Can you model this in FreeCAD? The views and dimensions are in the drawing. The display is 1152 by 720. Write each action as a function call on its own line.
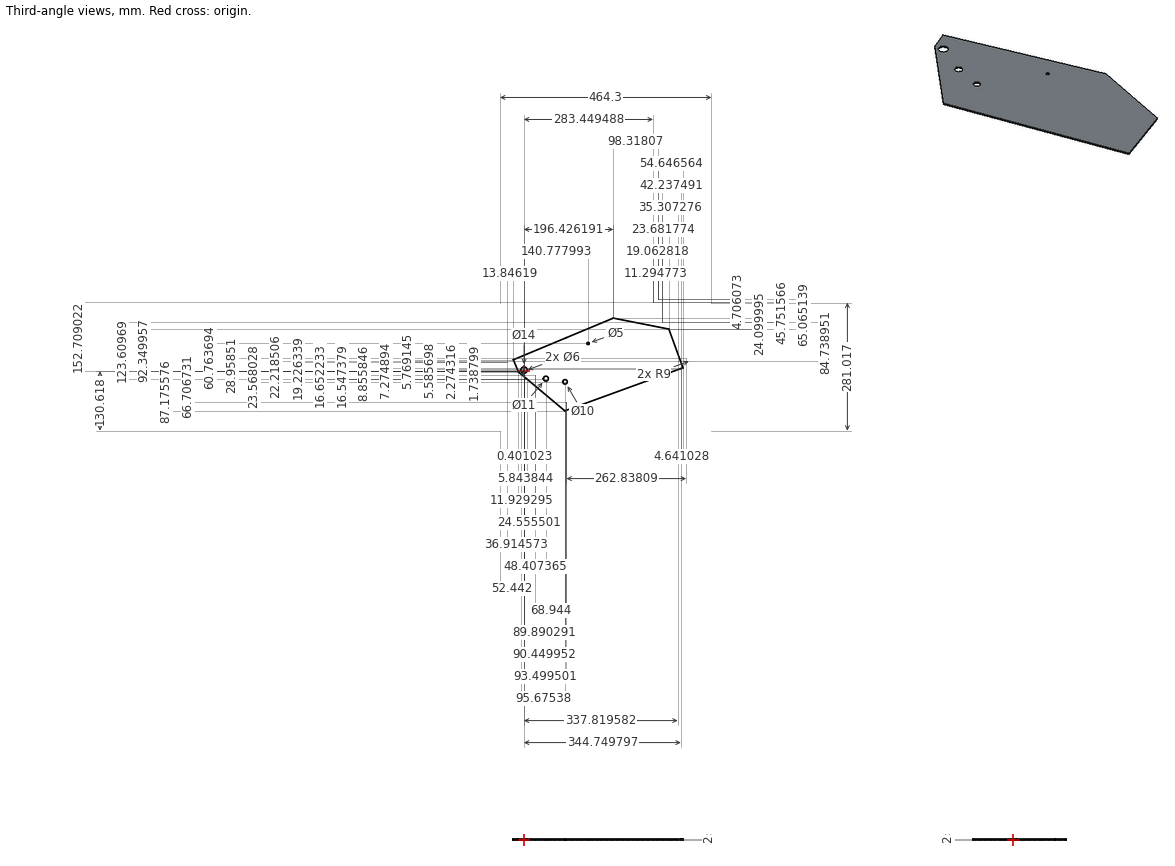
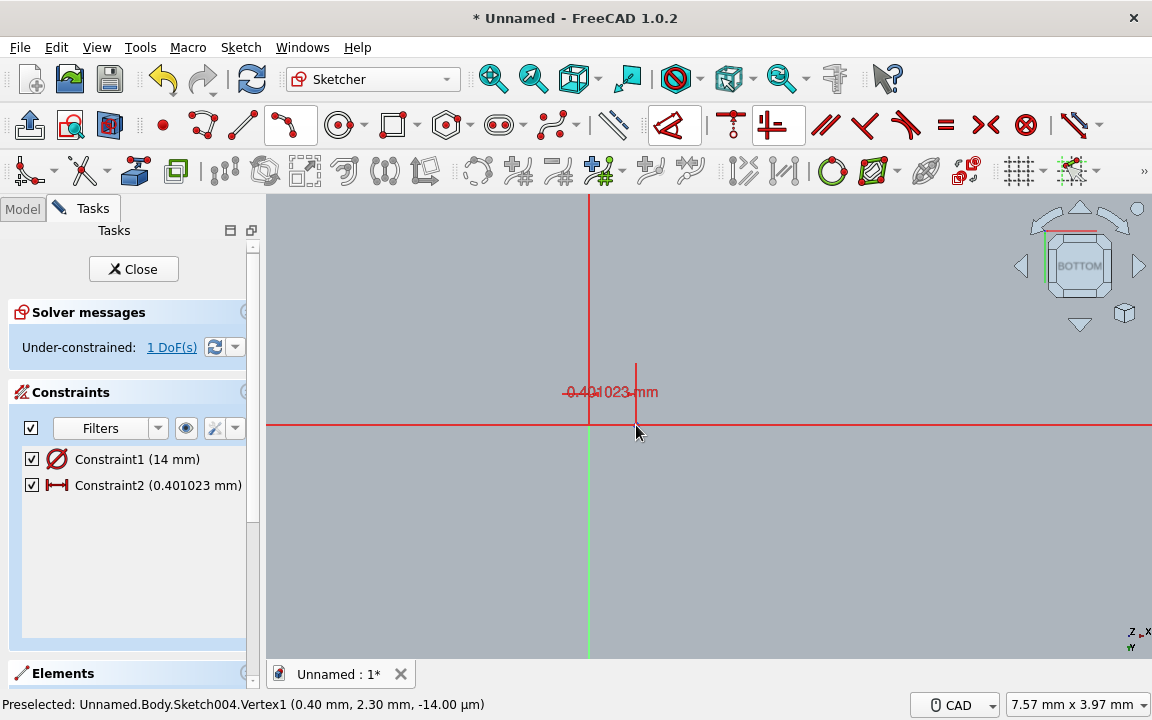
scroll(641, 427, down, 9)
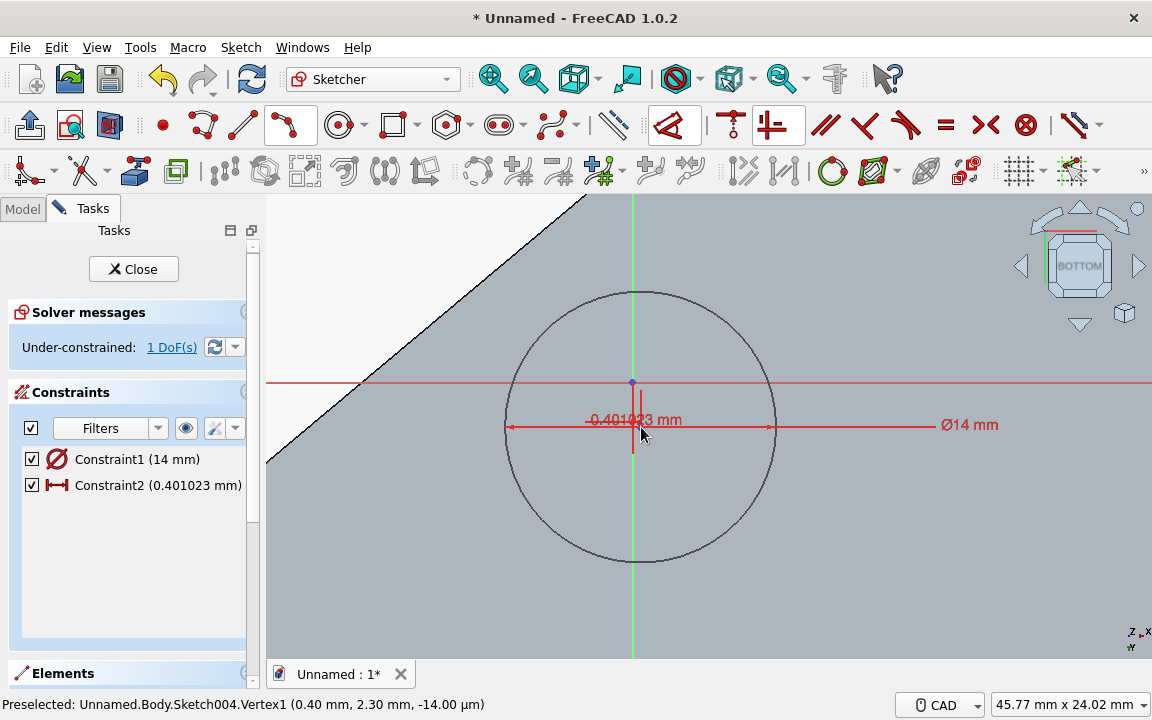
click(641, 427)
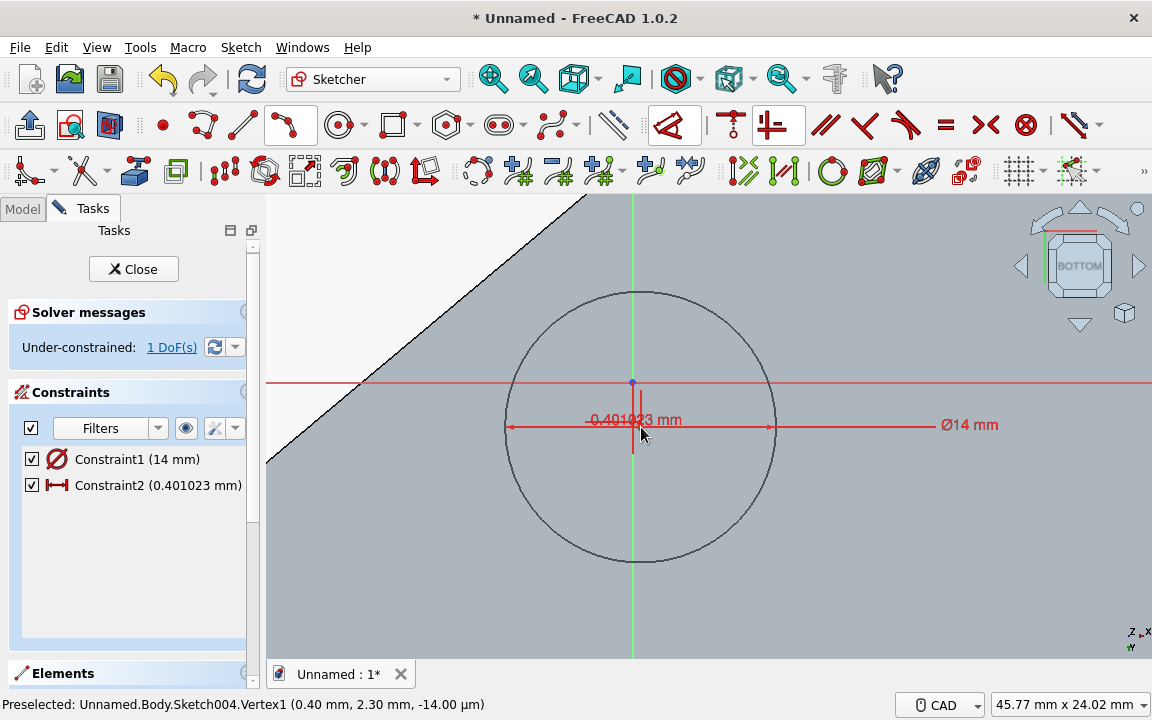
key(i)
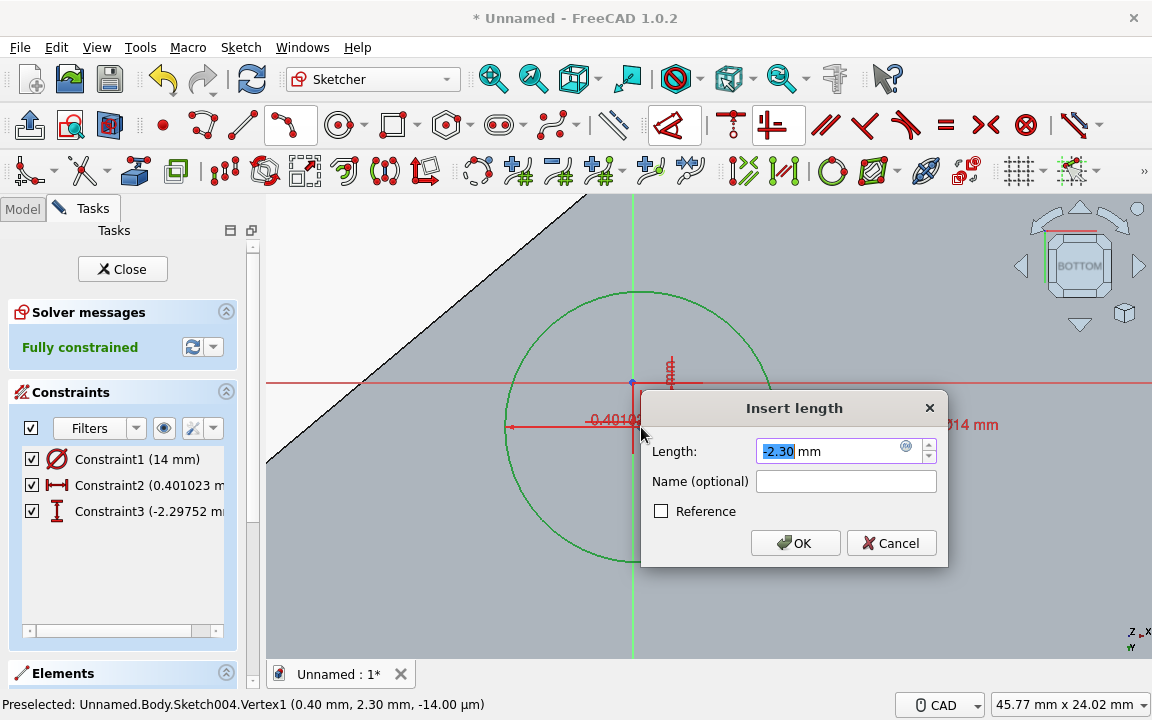
text(-2.274316)
key(Return)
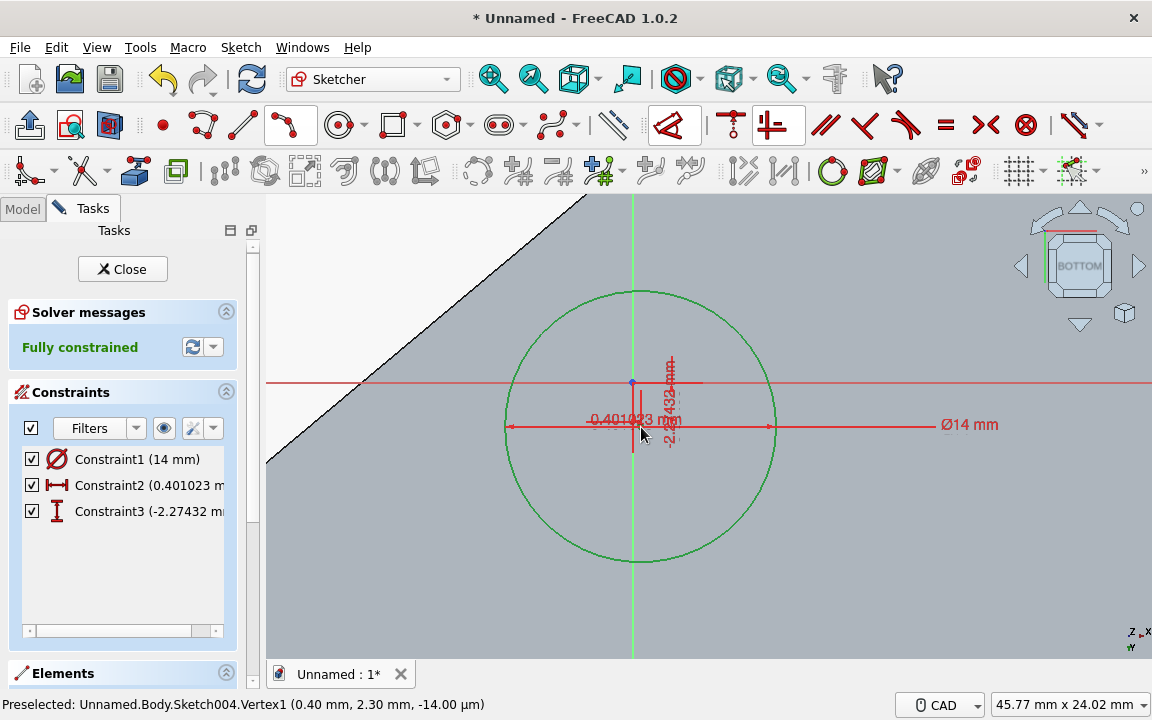
click(123, 269)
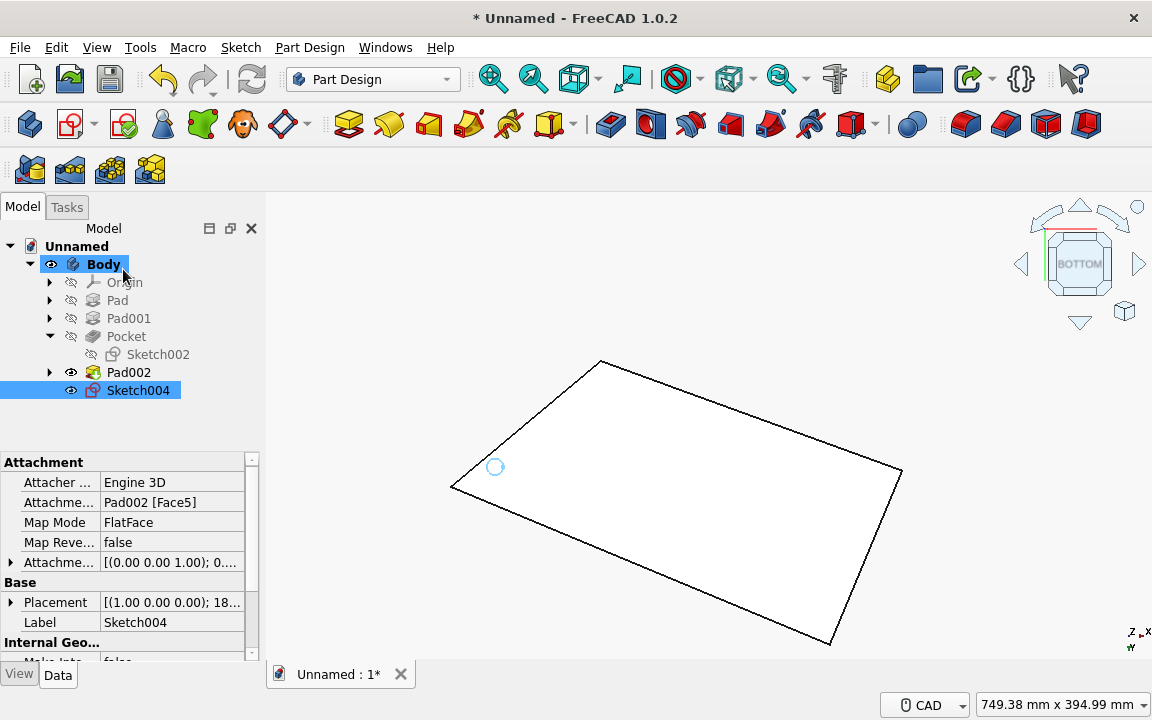
click(612, 124)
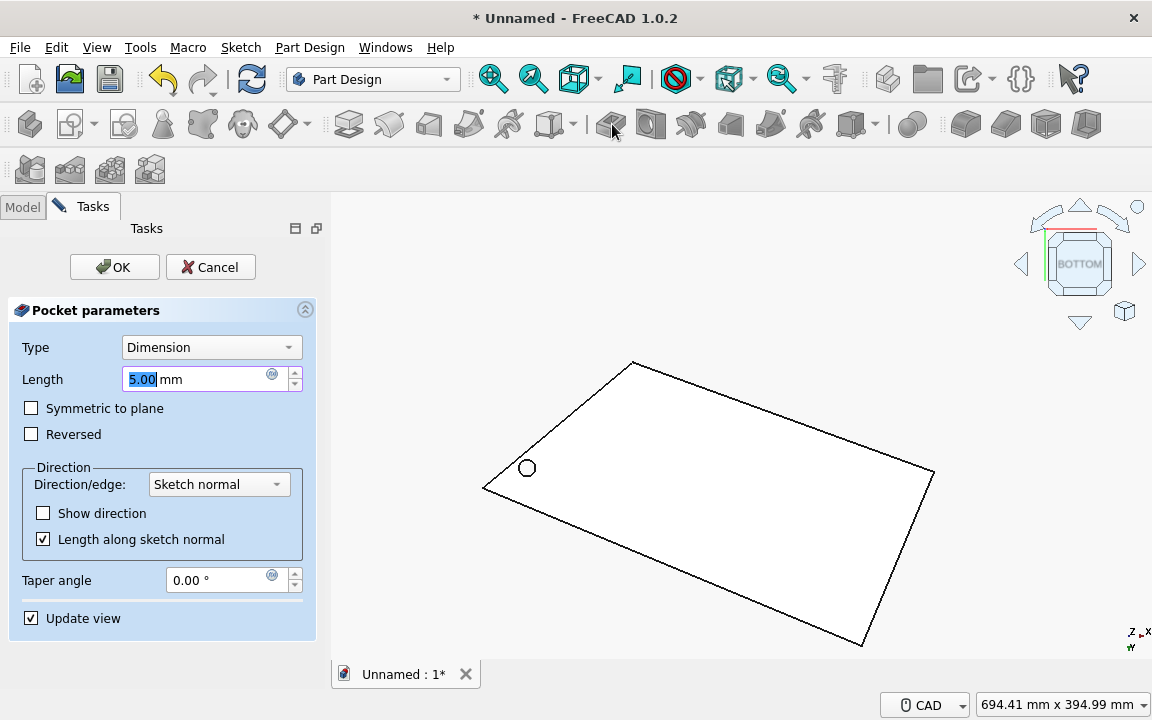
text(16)
key(Tab)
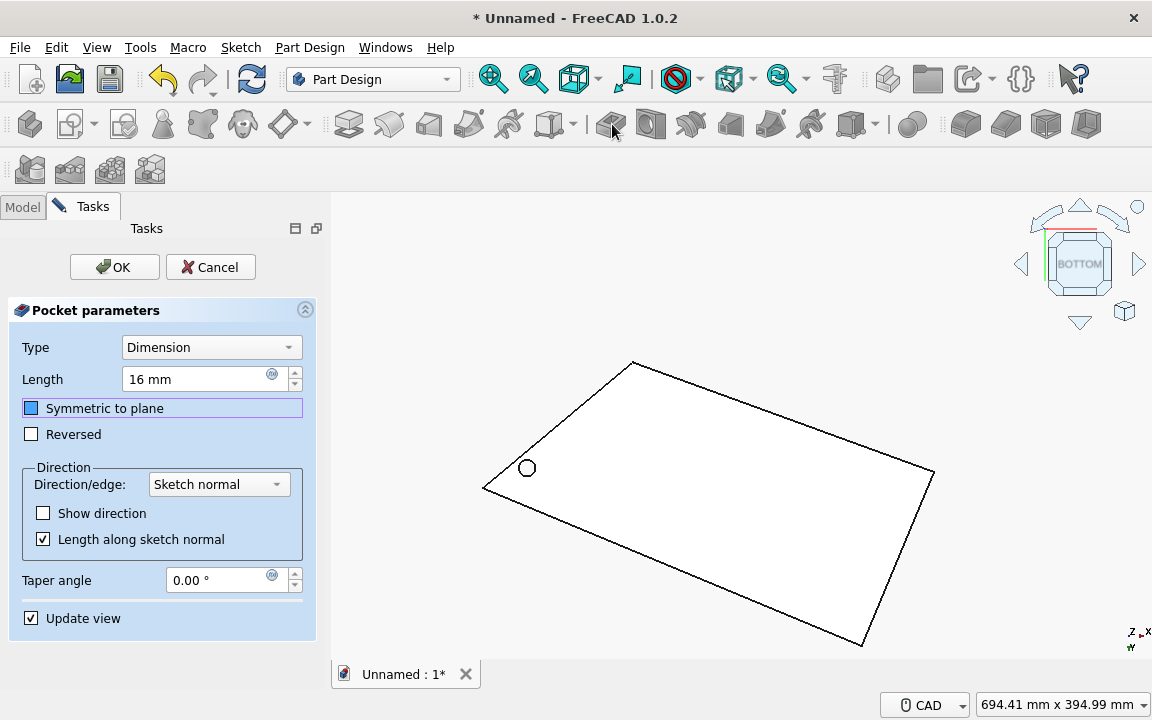
click(115, 267)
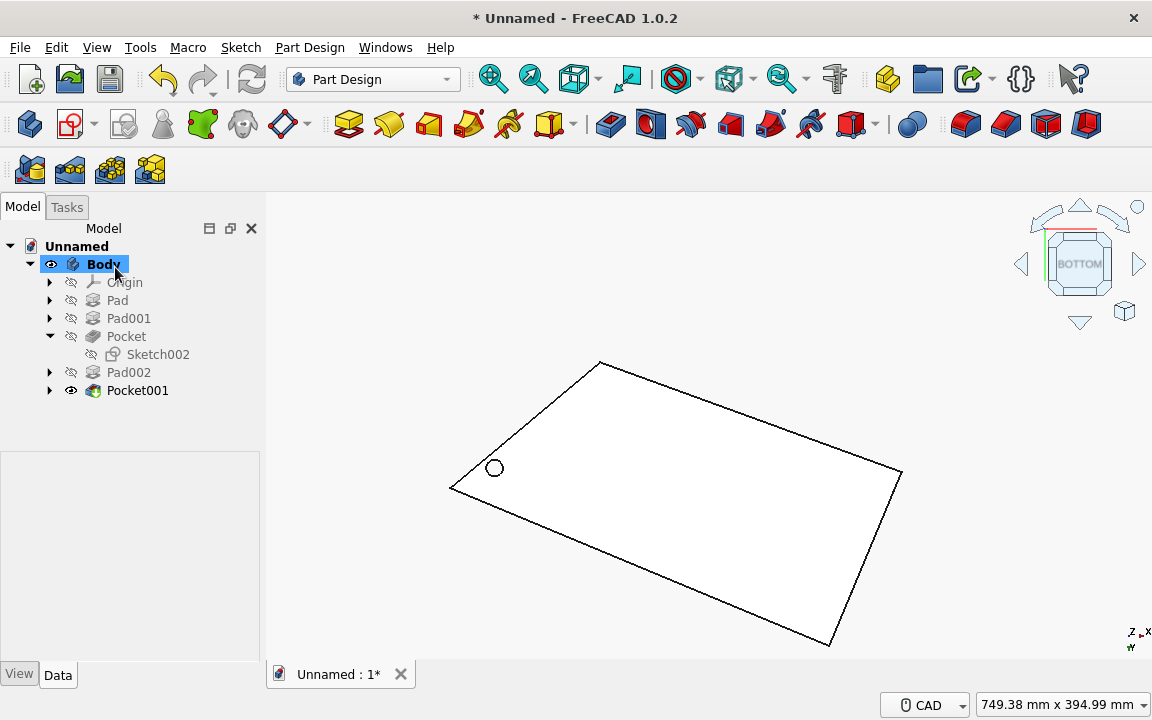
click(70, 124)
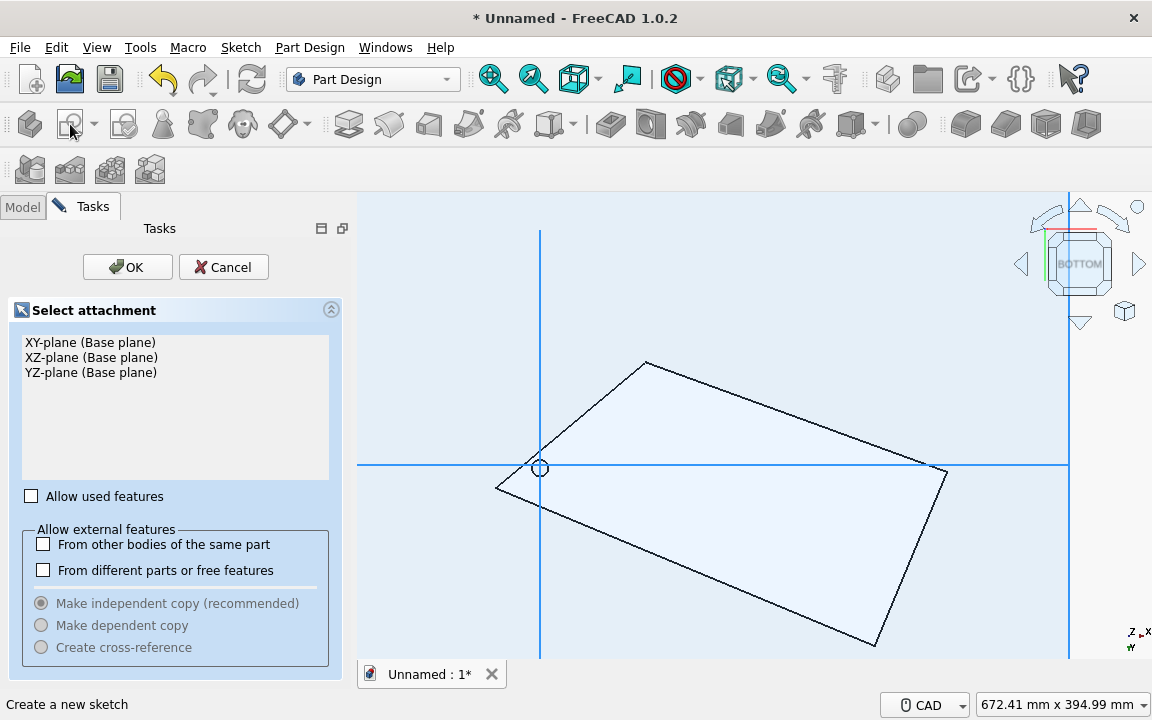
click(82, 342)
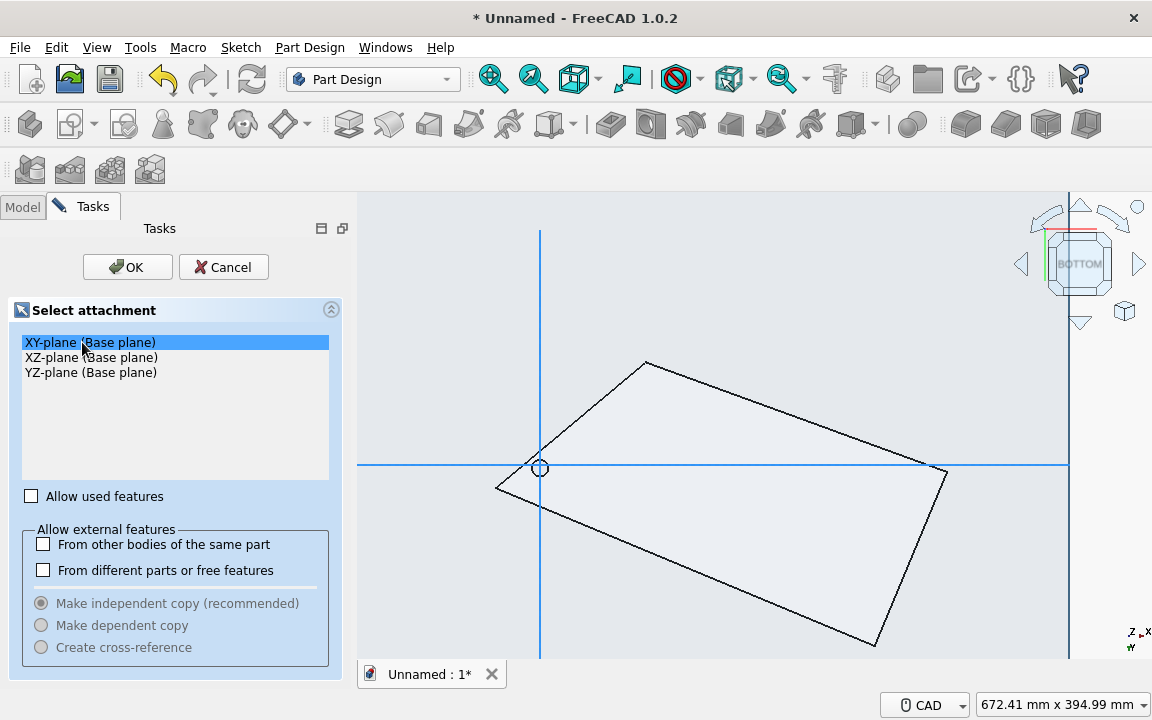
click(128, 267)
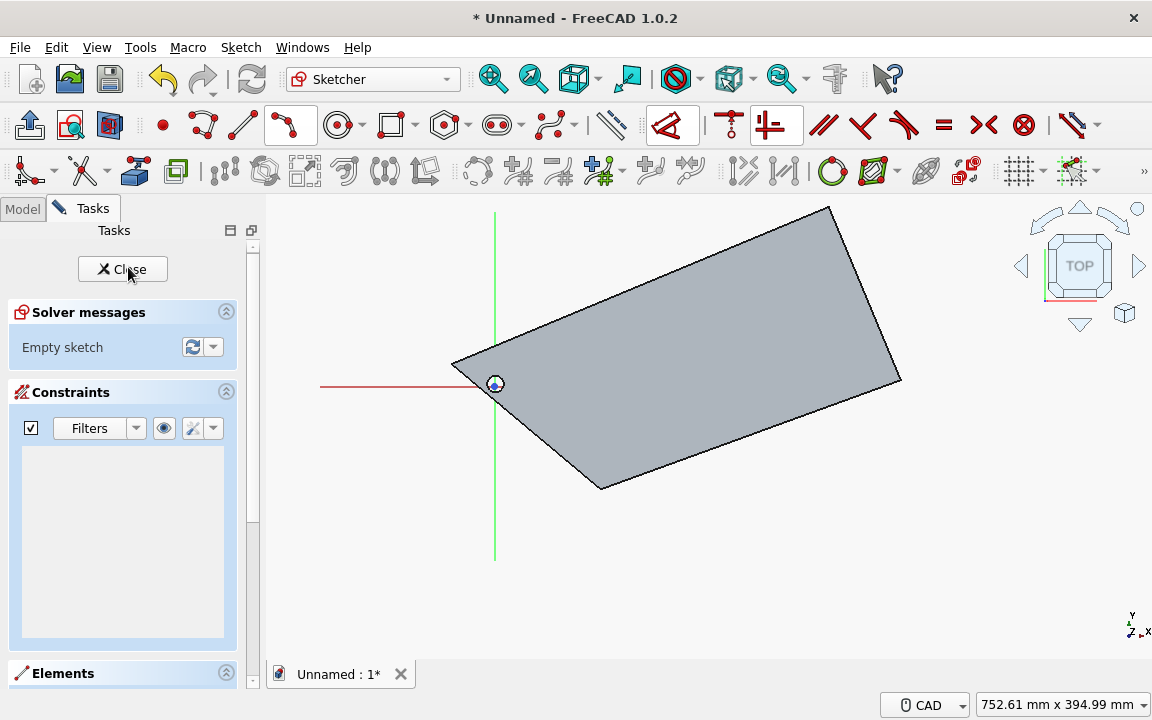
click(110, 126)